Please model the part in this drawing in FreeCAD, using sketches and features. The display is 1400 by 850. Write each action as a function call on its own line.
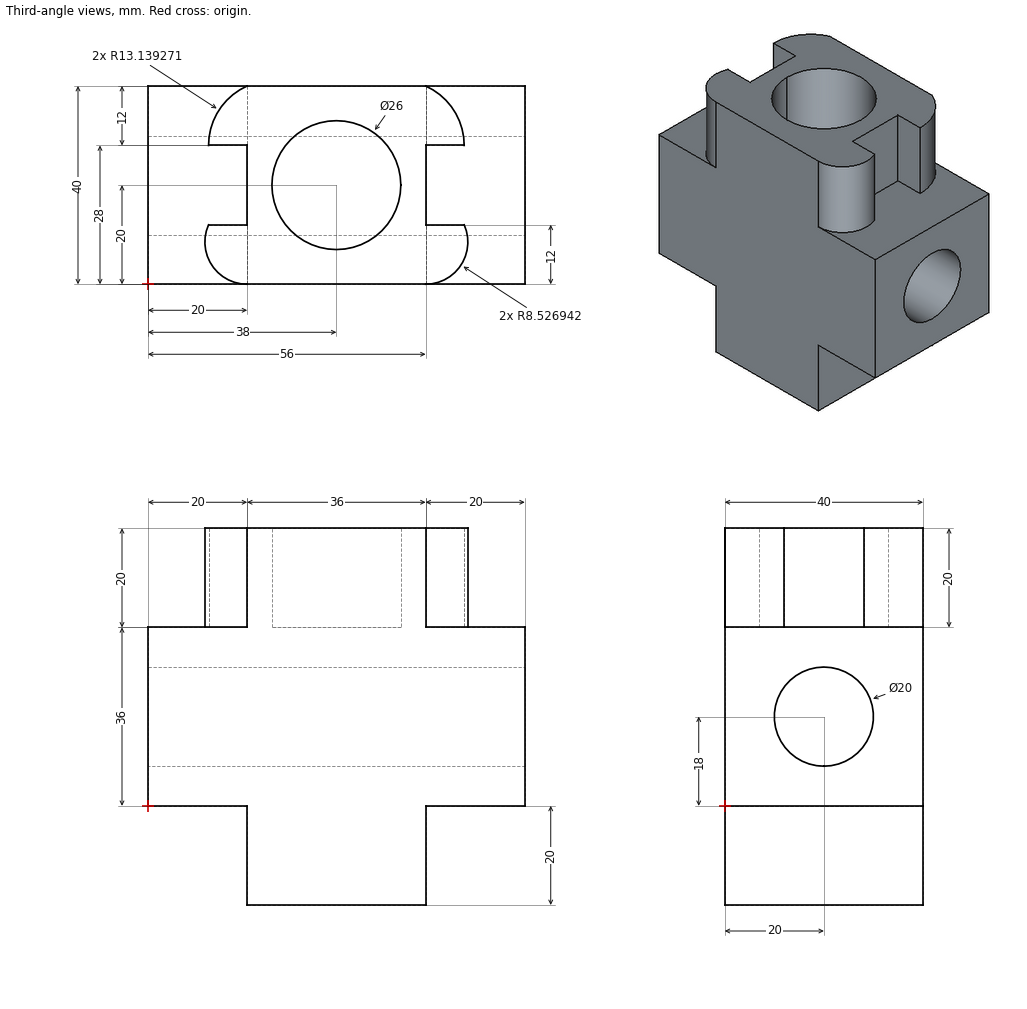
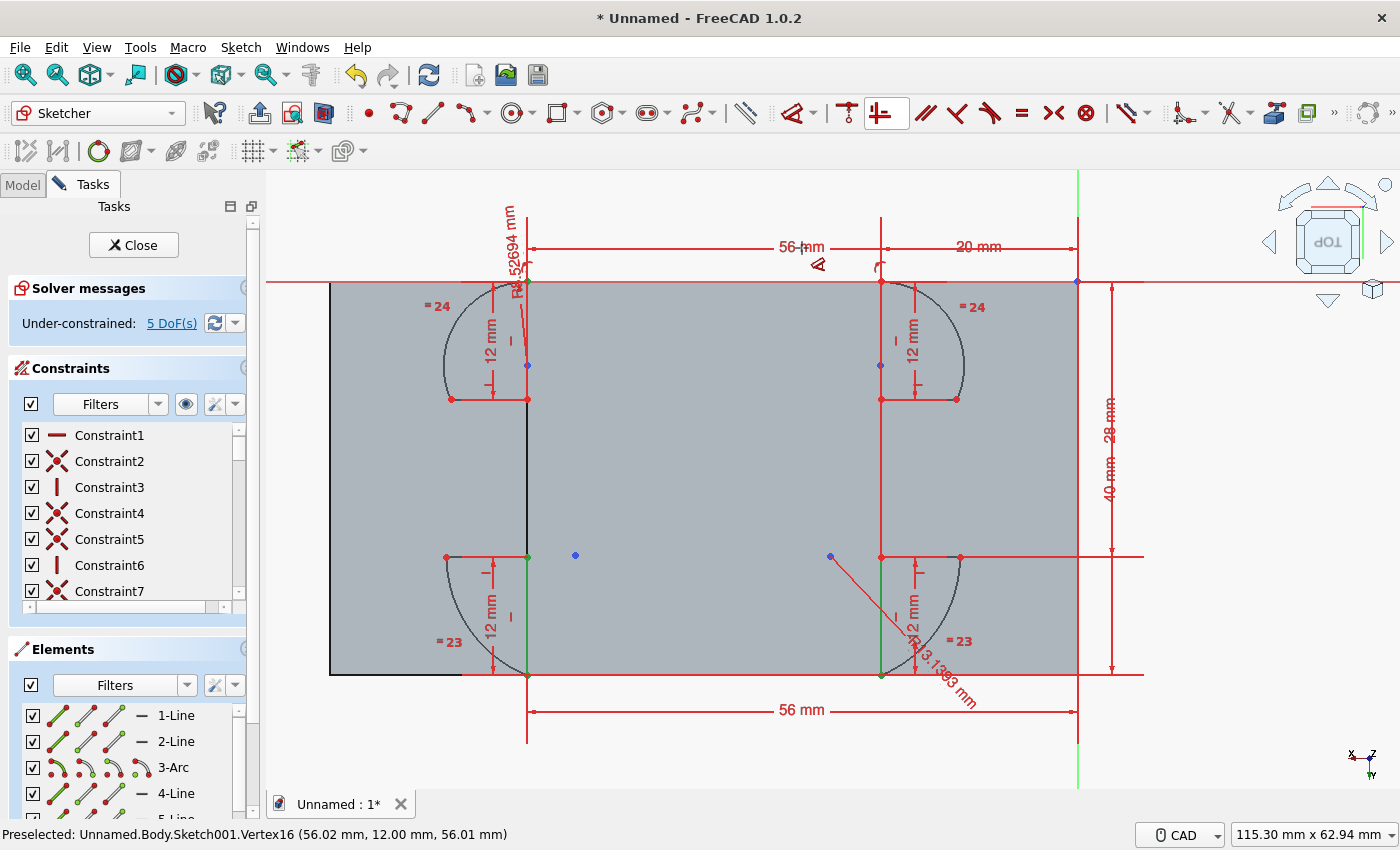
click(881, 282)
click(979, 316)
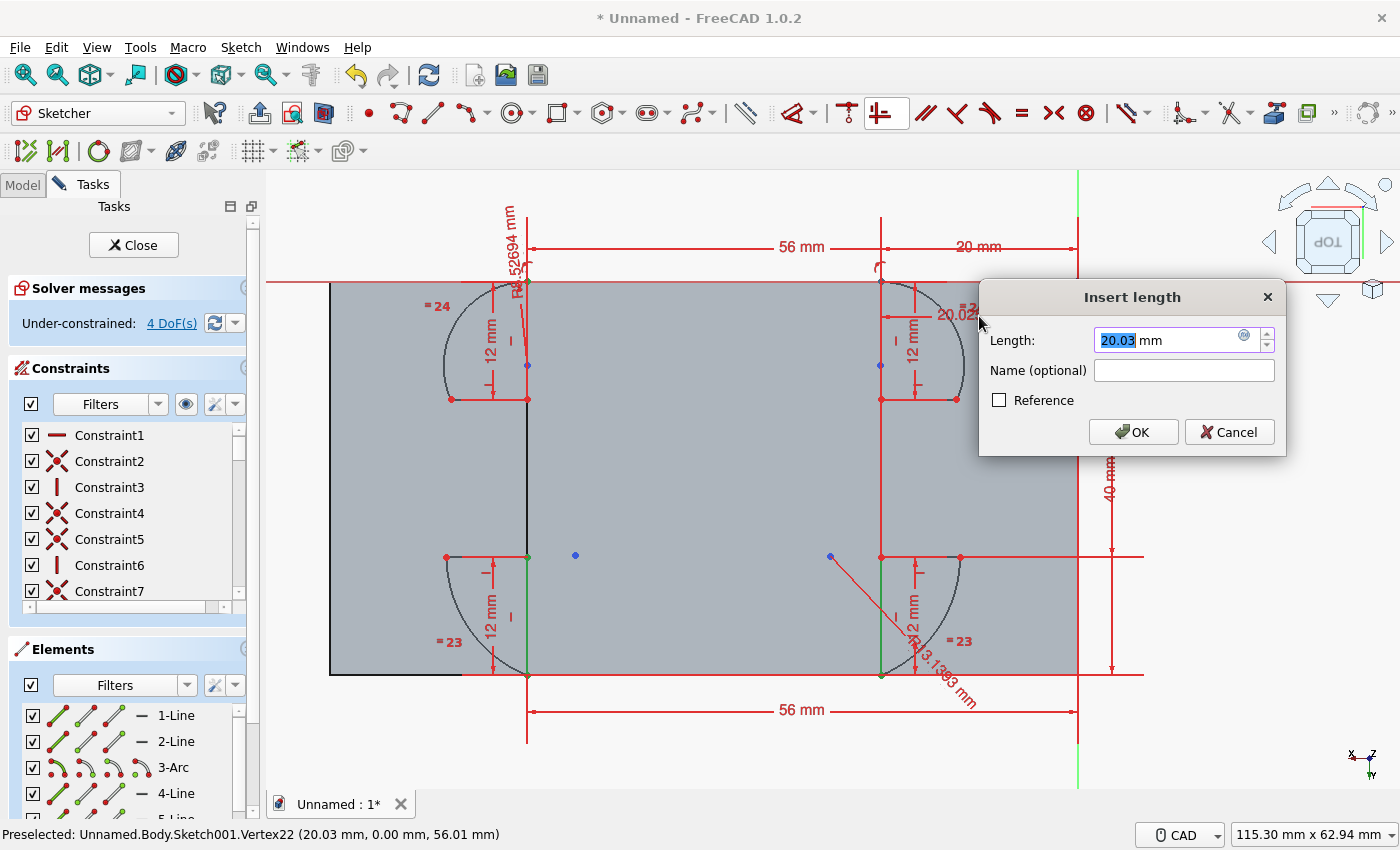
text(20)
key(Return)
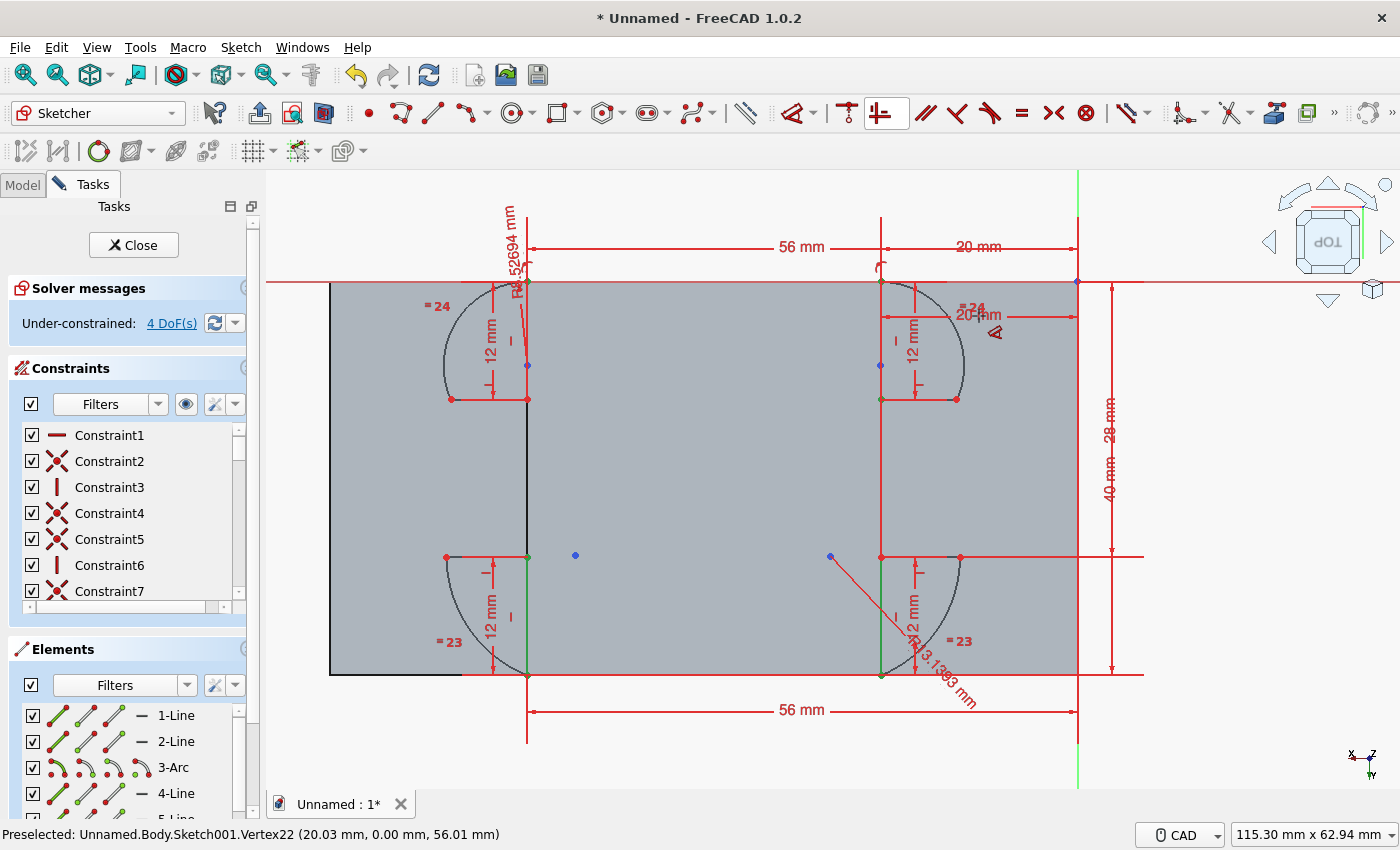
click(831, 556)
click(1112, 356)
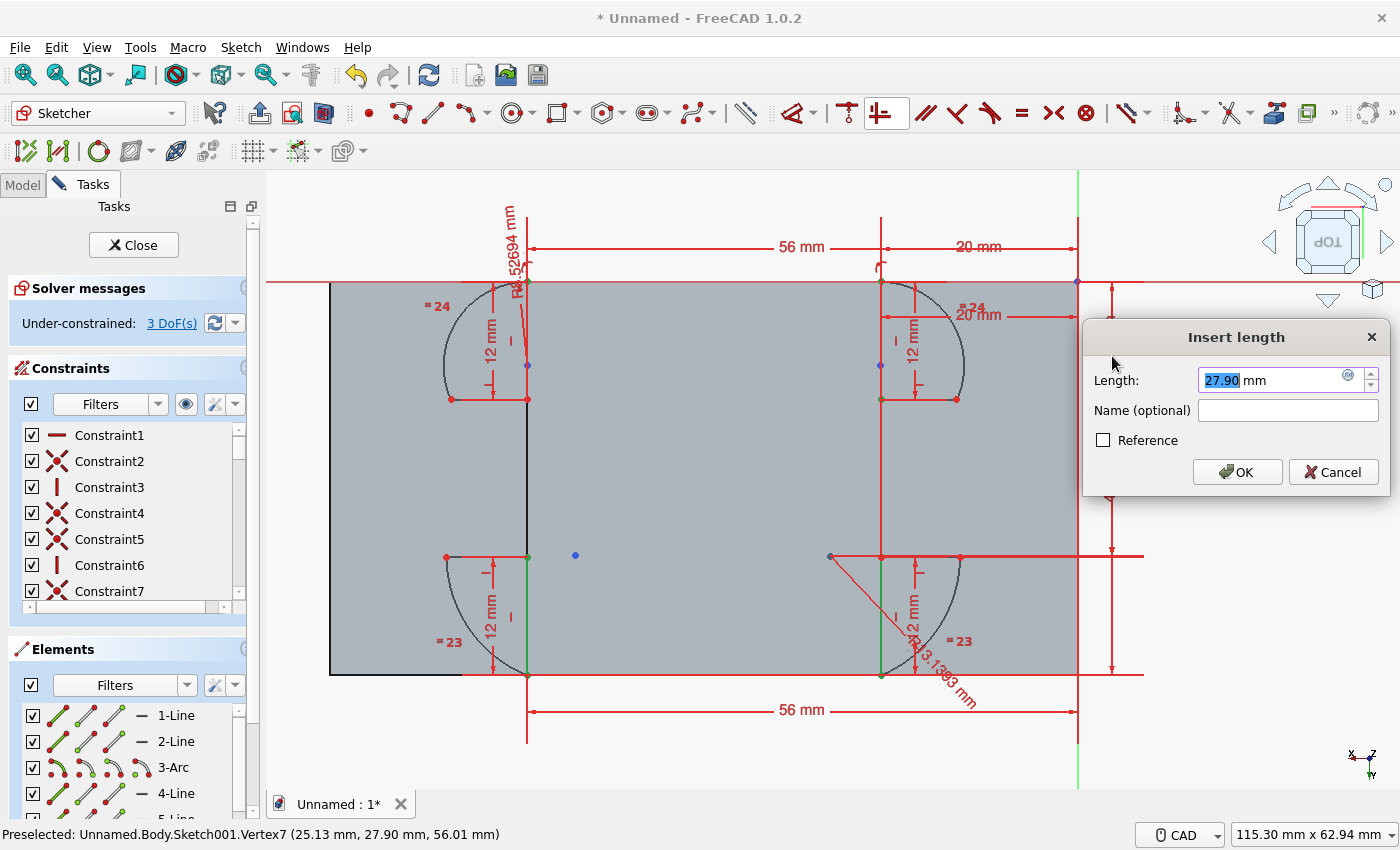
text(28)
key(Return)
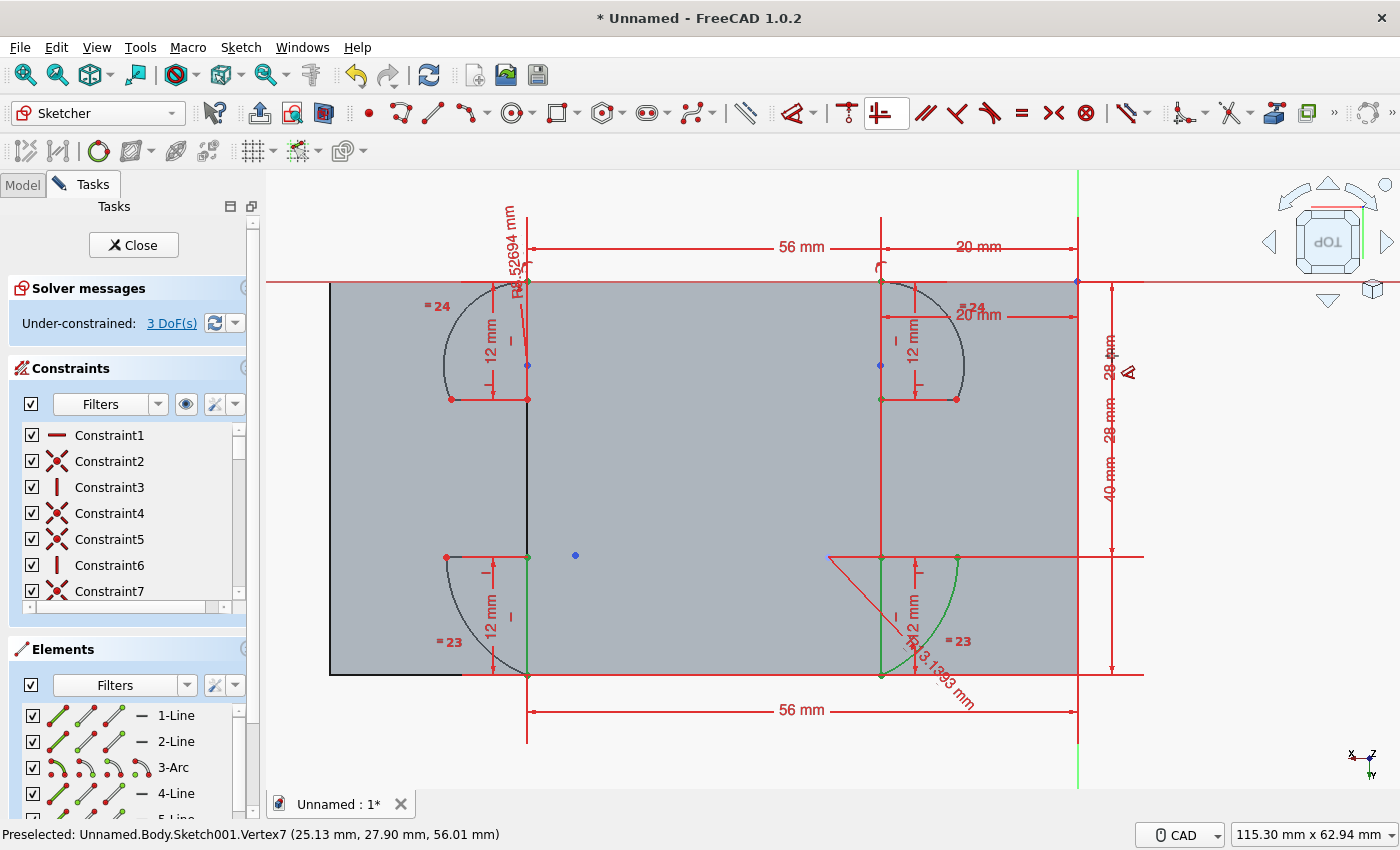
click(576, 556)
click(1112, 323)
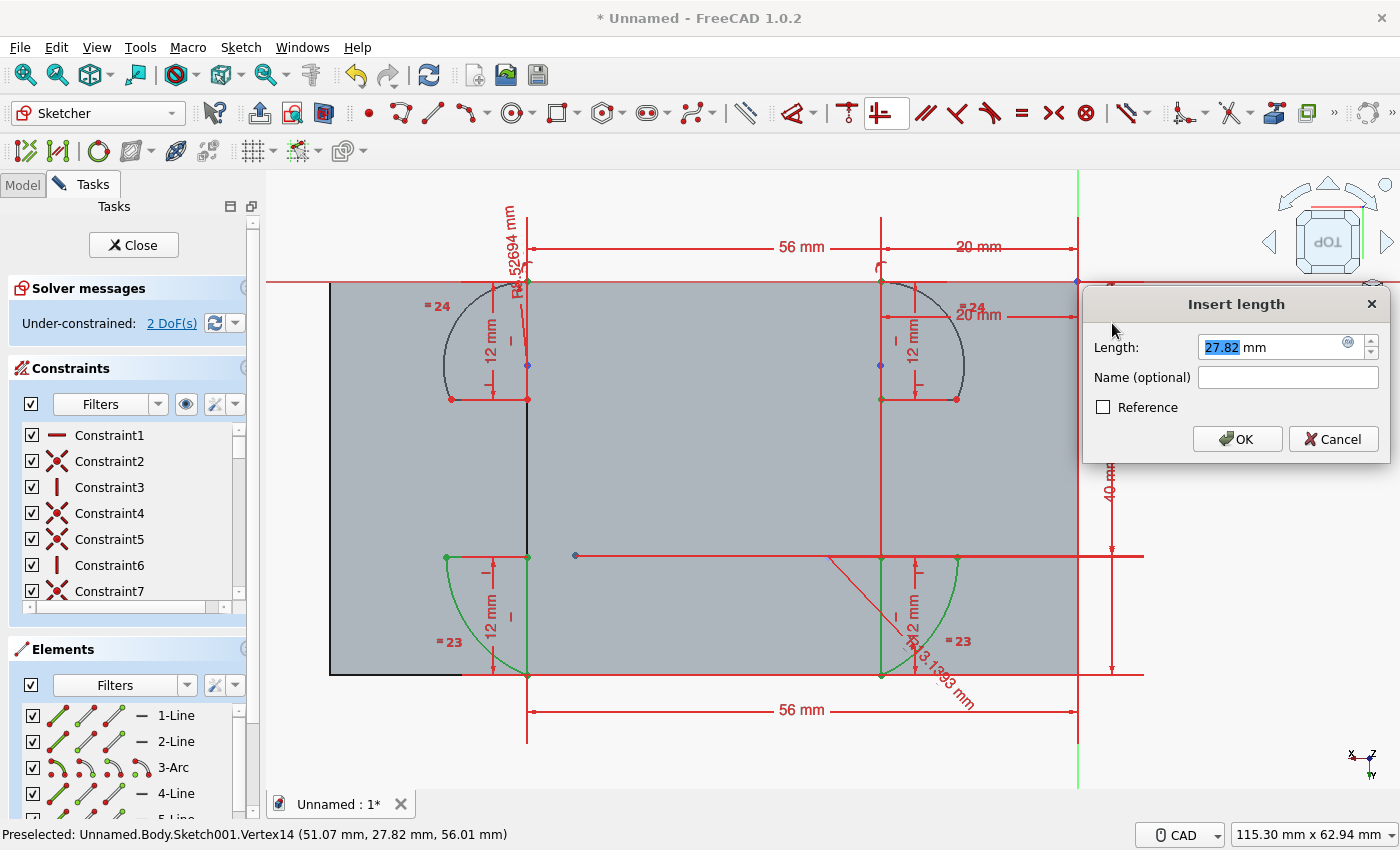
text(28)
key(Return)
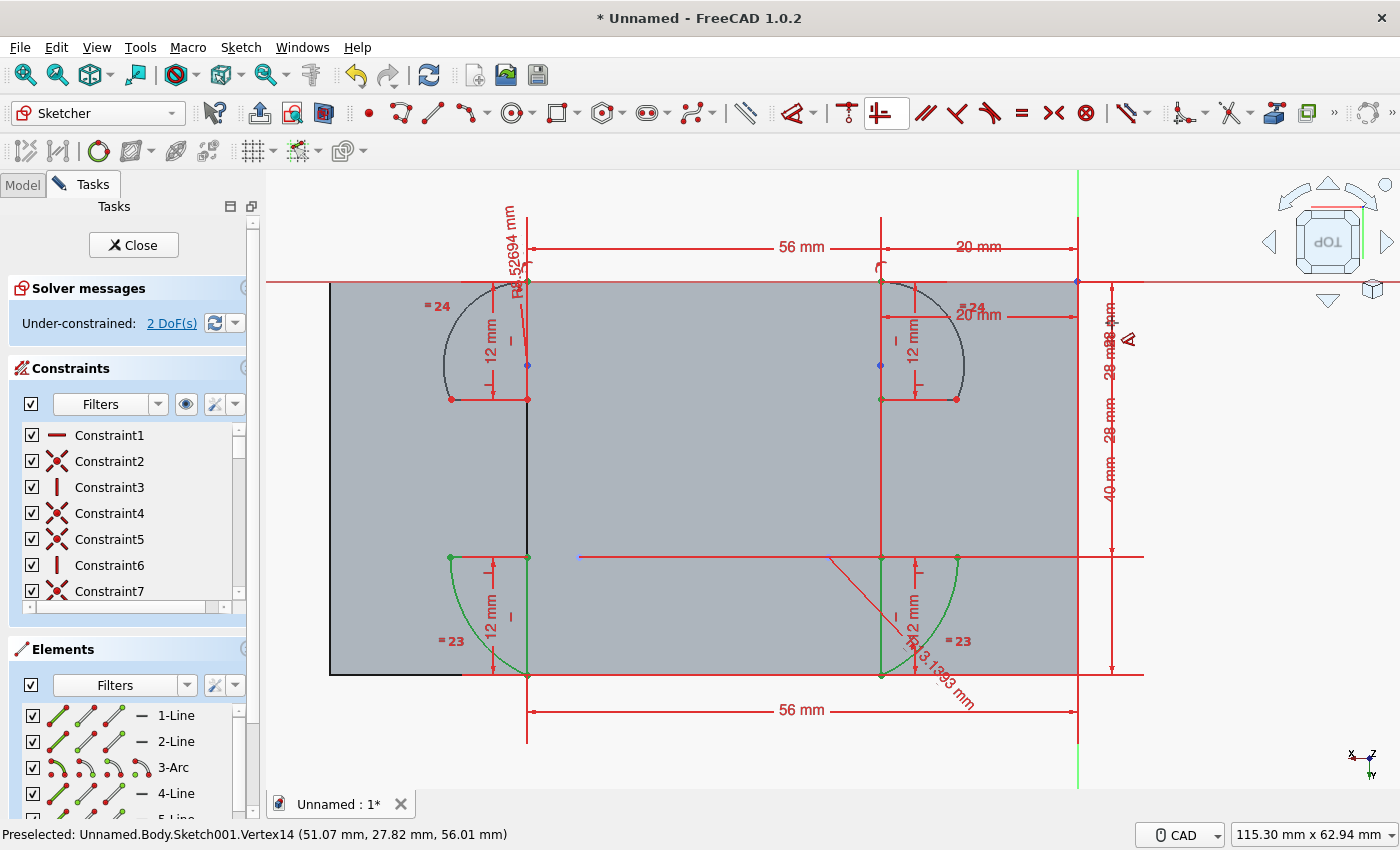
click(528, 366)
click(676, 248)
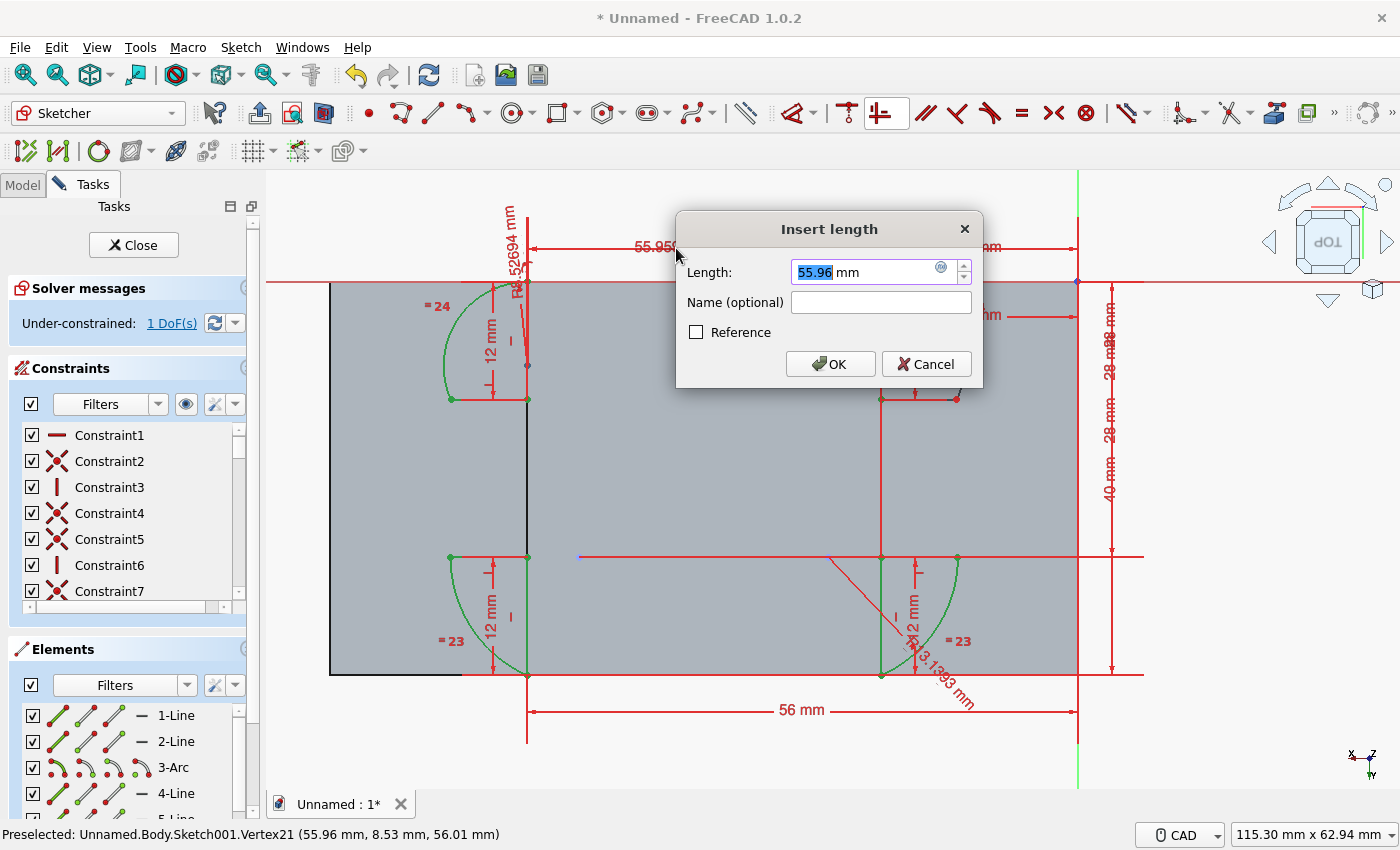
text(56)
key(Return)